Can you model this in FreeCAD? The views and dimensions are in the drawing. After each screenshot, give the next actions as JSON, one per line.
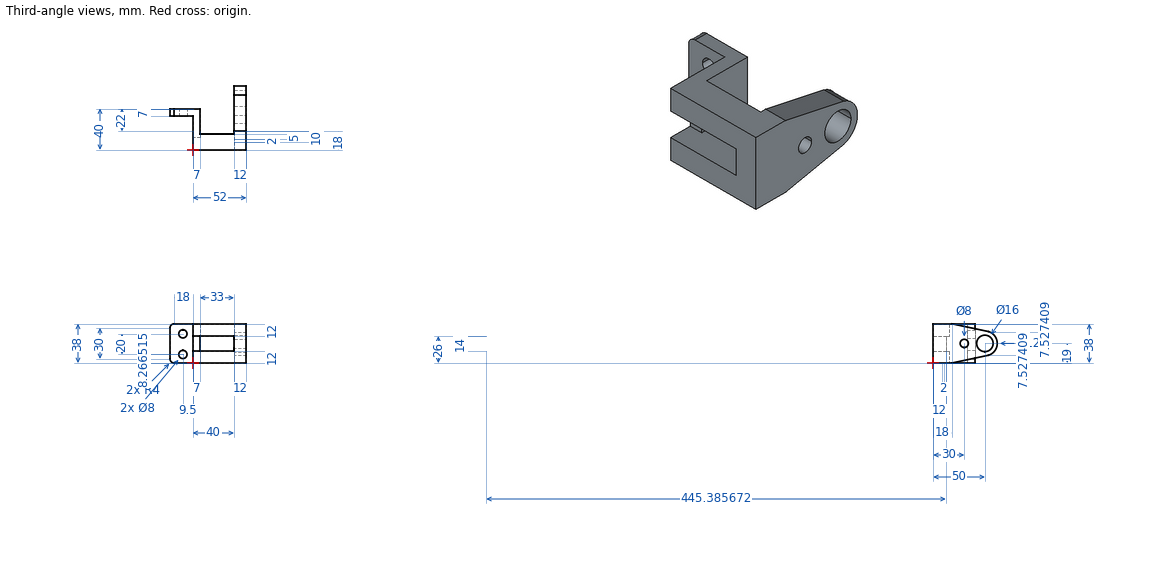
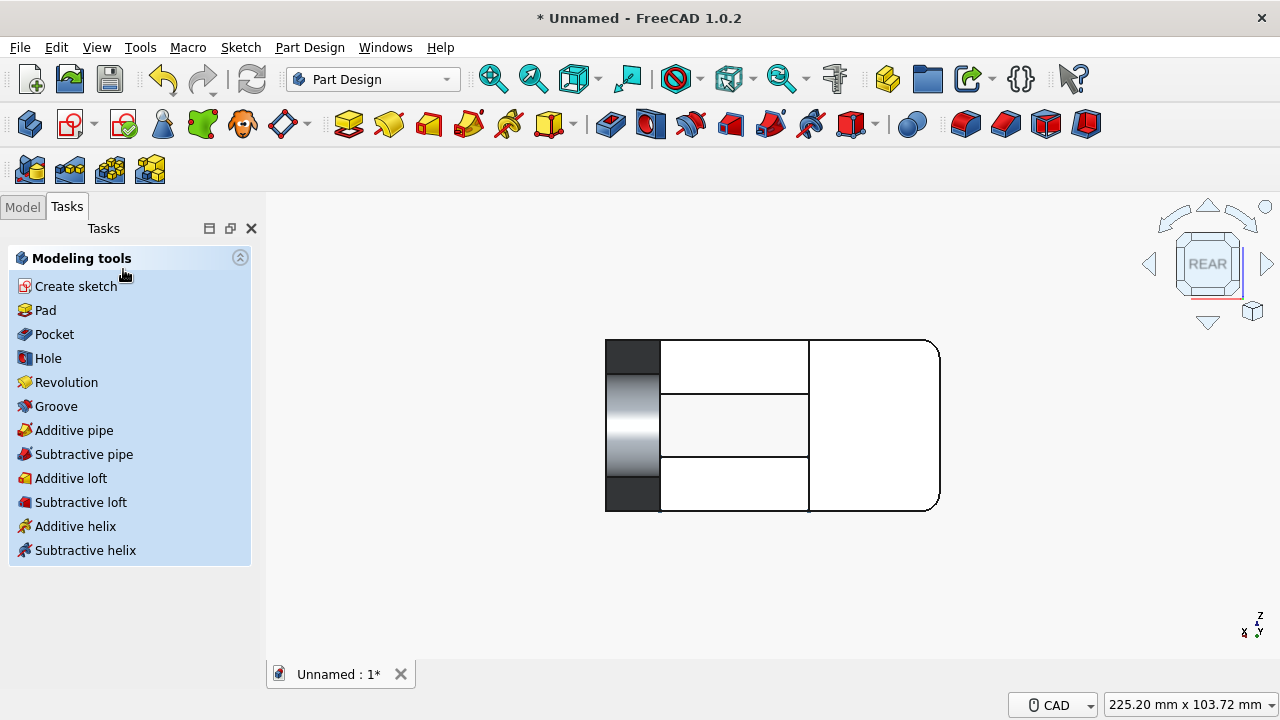
{"action": "left_click", "coordinate": [350, 124]}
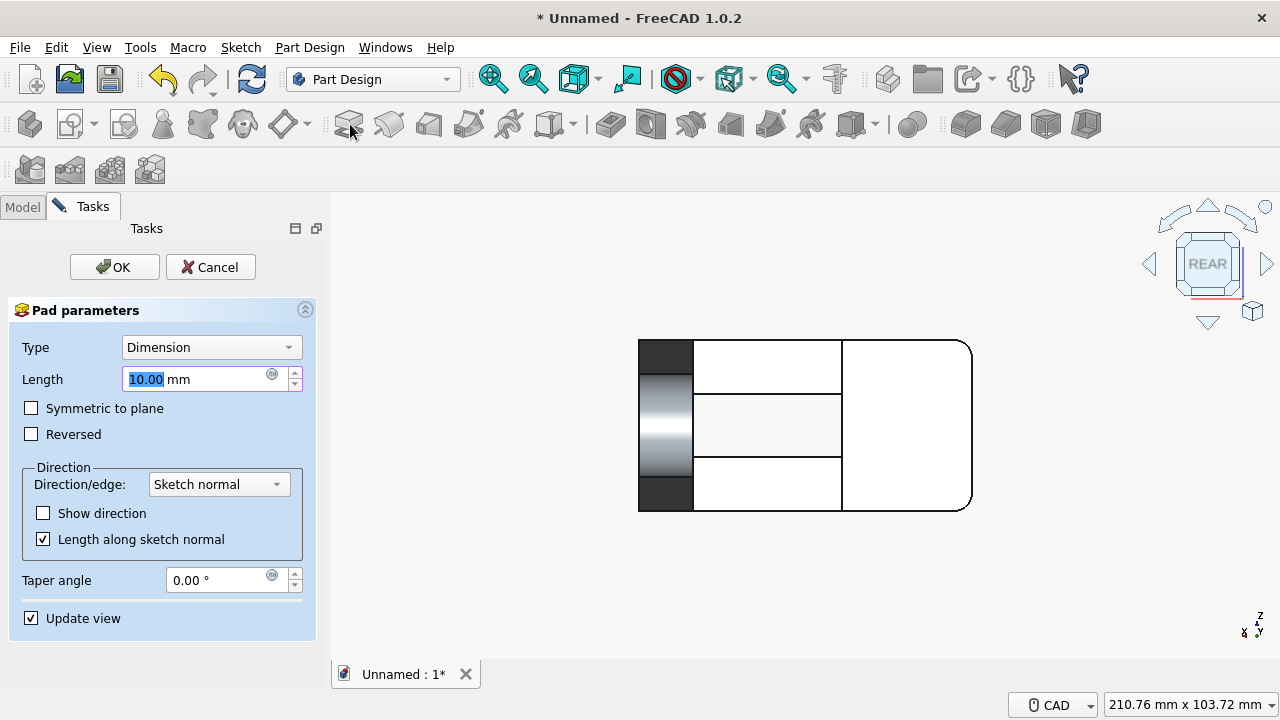
{"action": "type", "text": "2"}
{"action": "key", "text": "Tab"}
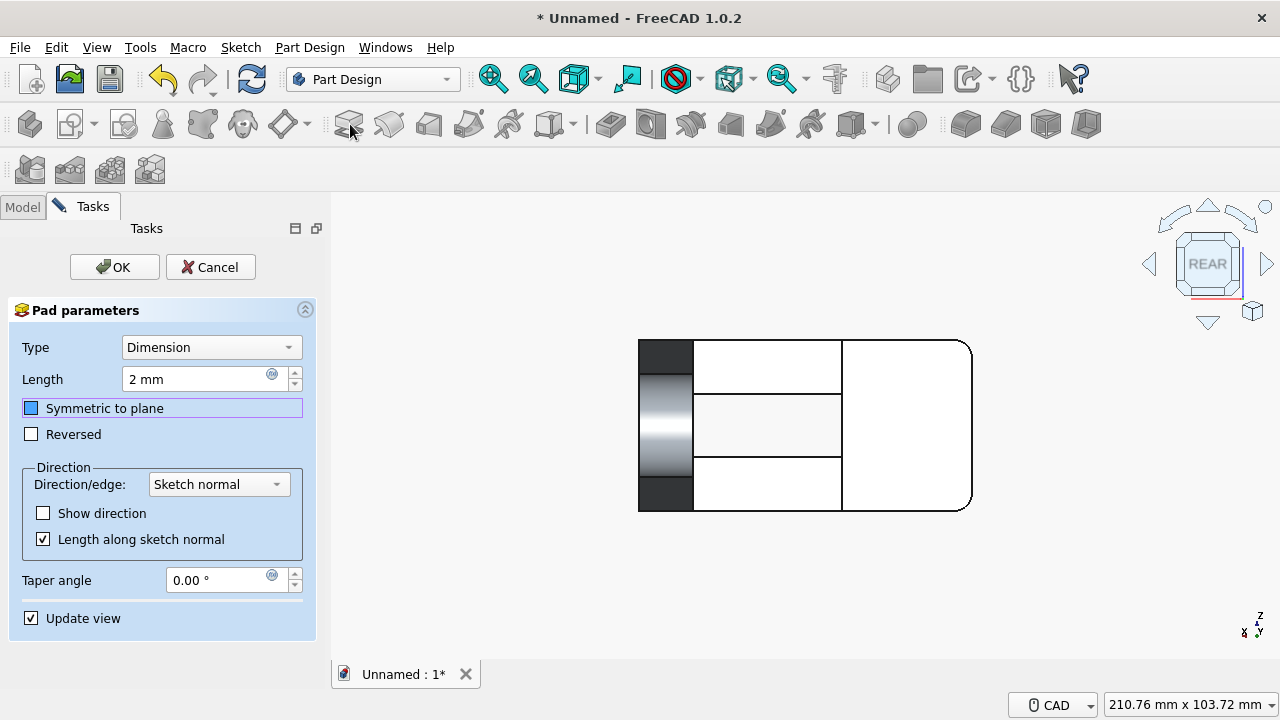
{"action": "left_click", "coordinate": [115, 267]}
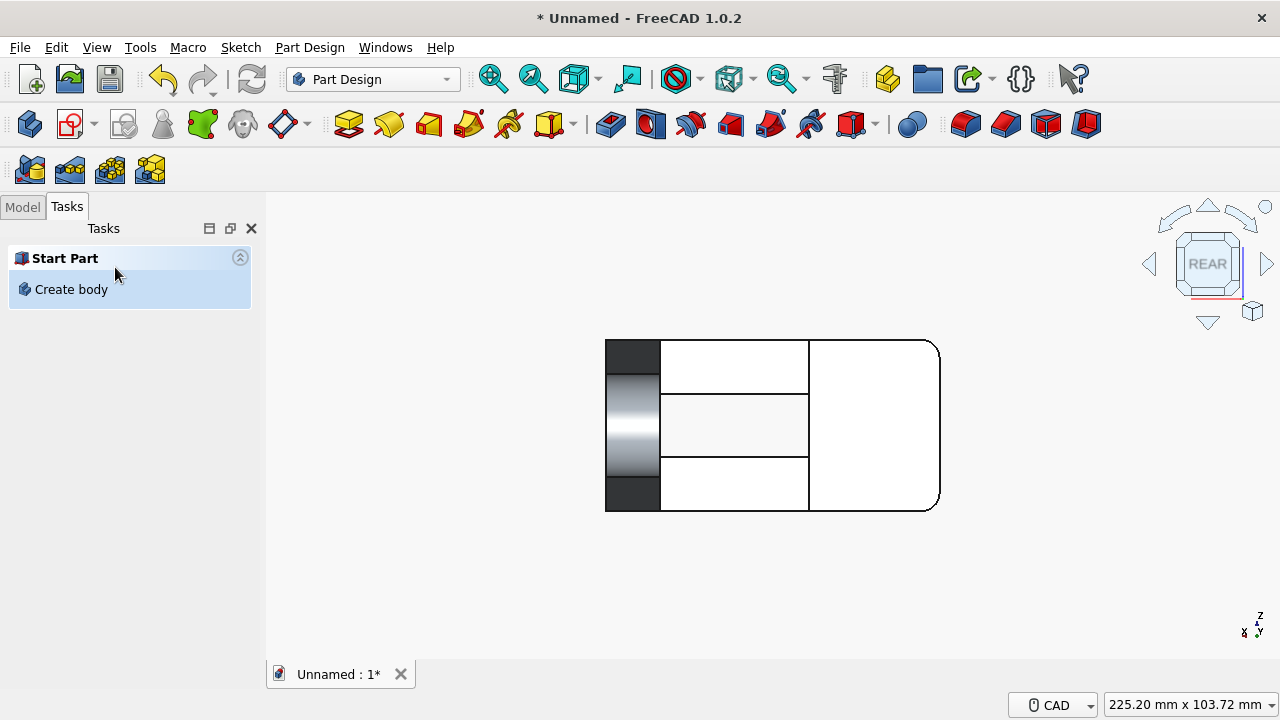
{"action": "left_click", "coordinate": [494, 80]}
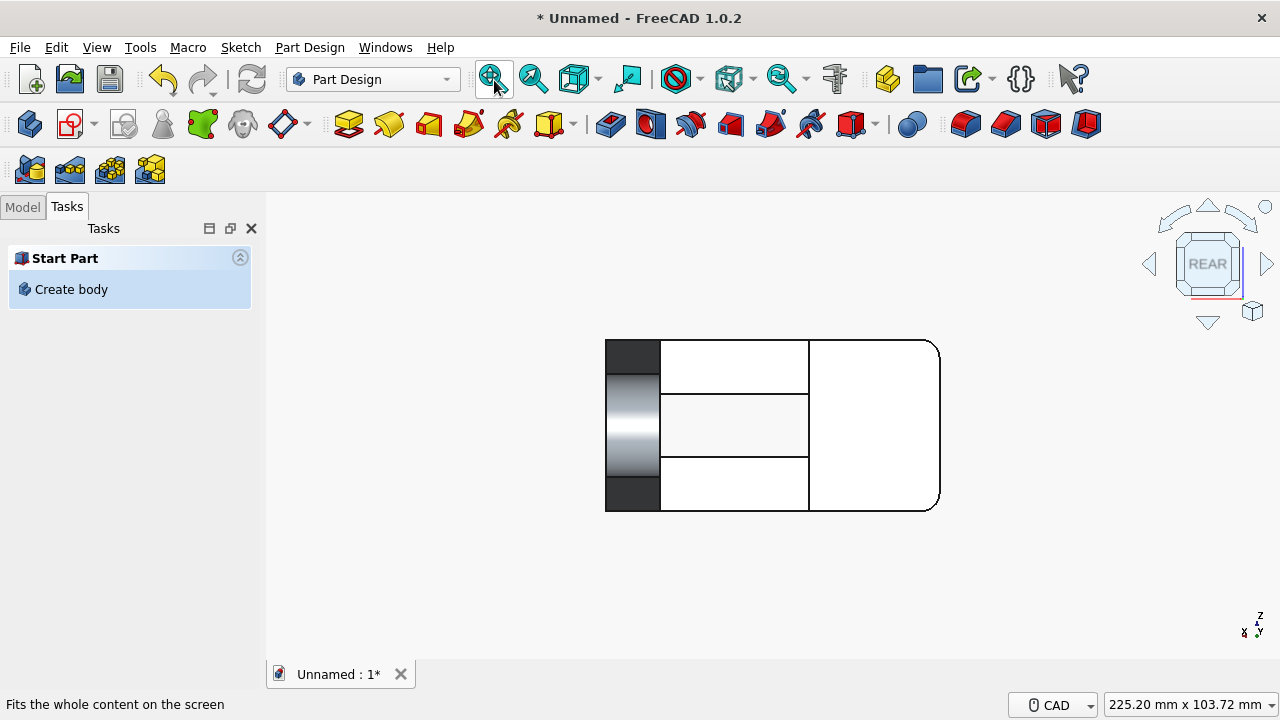
{"action": "left_click", "coordinate": [874, 424]}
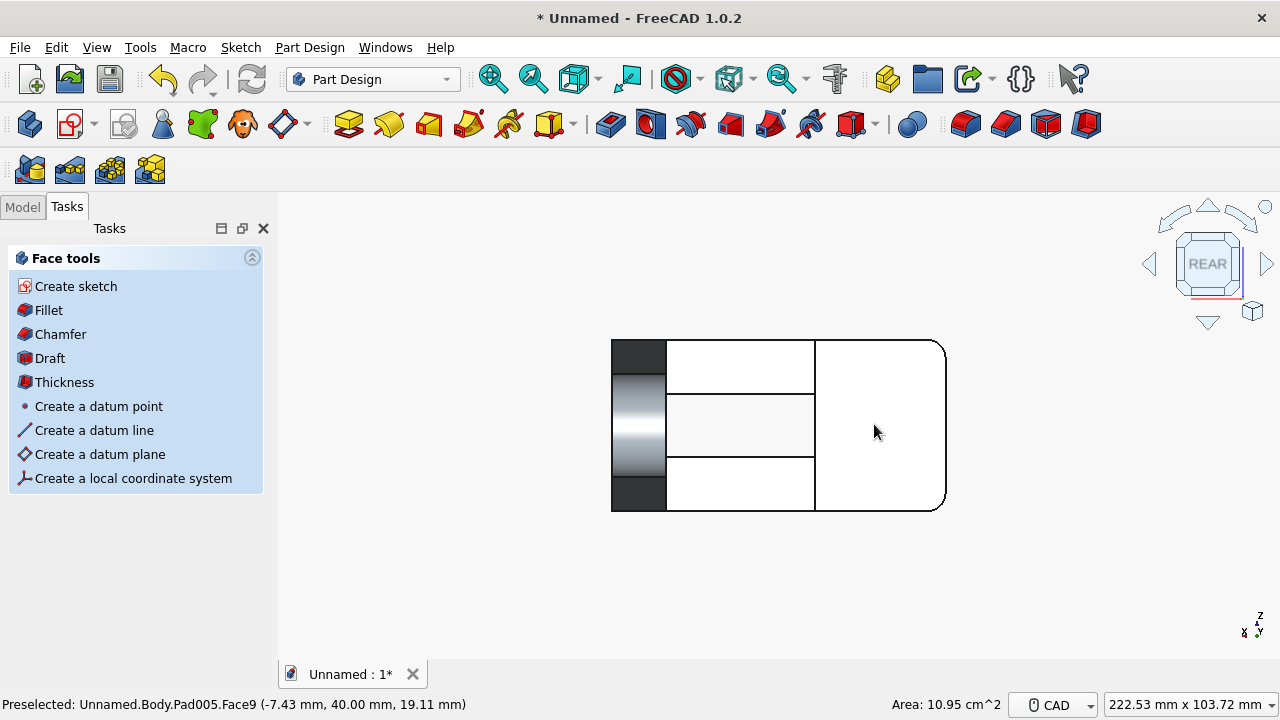
{"action": "left_click", "coordinate": [70, 124]}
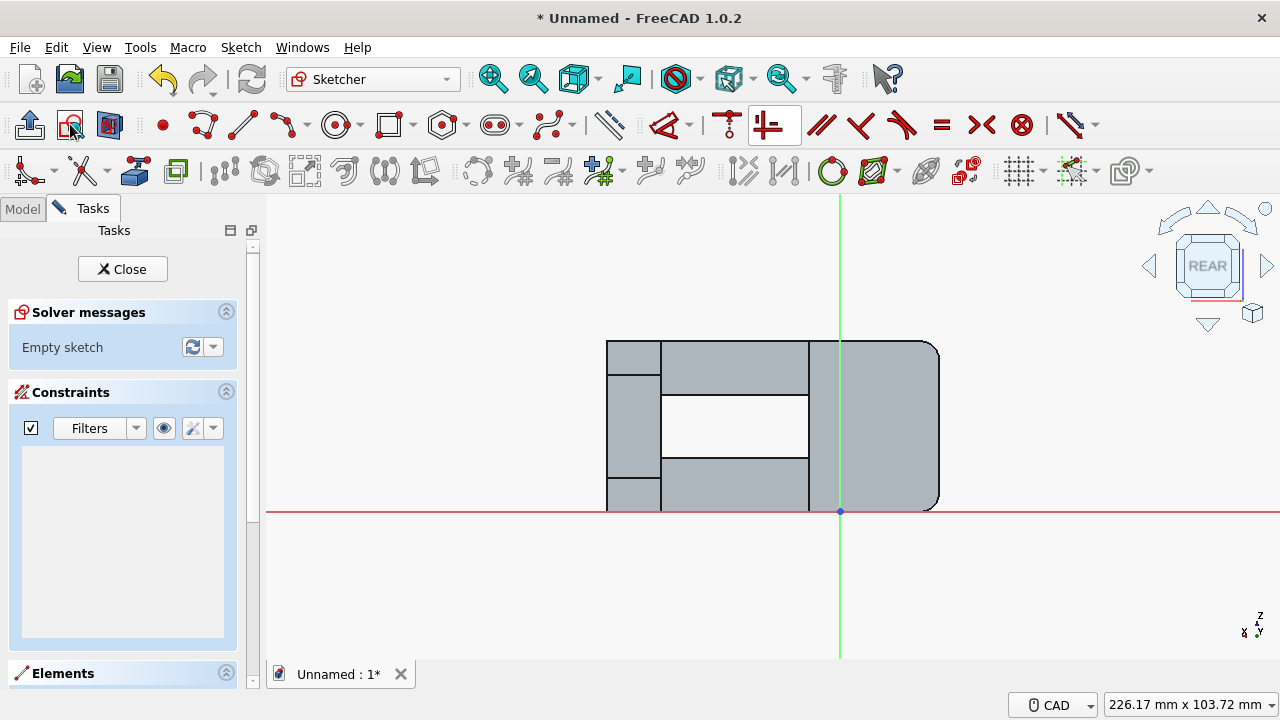
{"action": "left_click", "coordinate": [110, 126]}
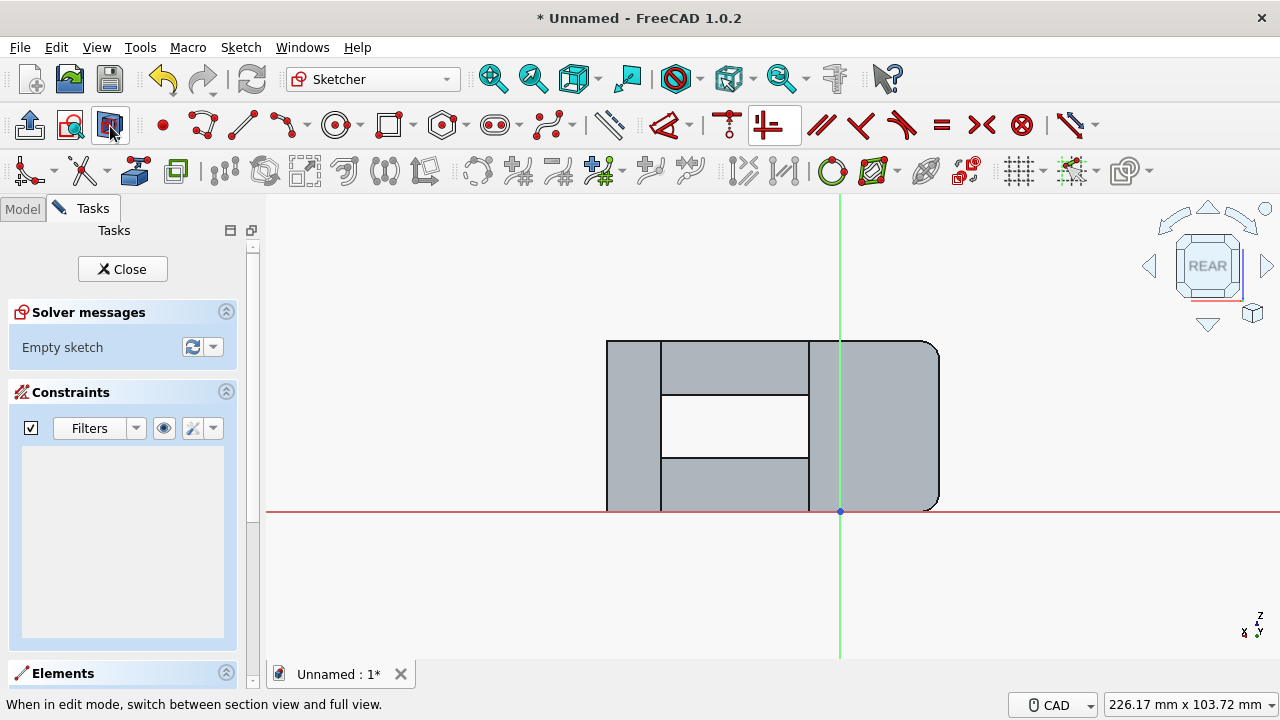
{"action": "scroll", "coordinate": [1072, 455], "scroll_direction": "up", "scroll_amount": 3}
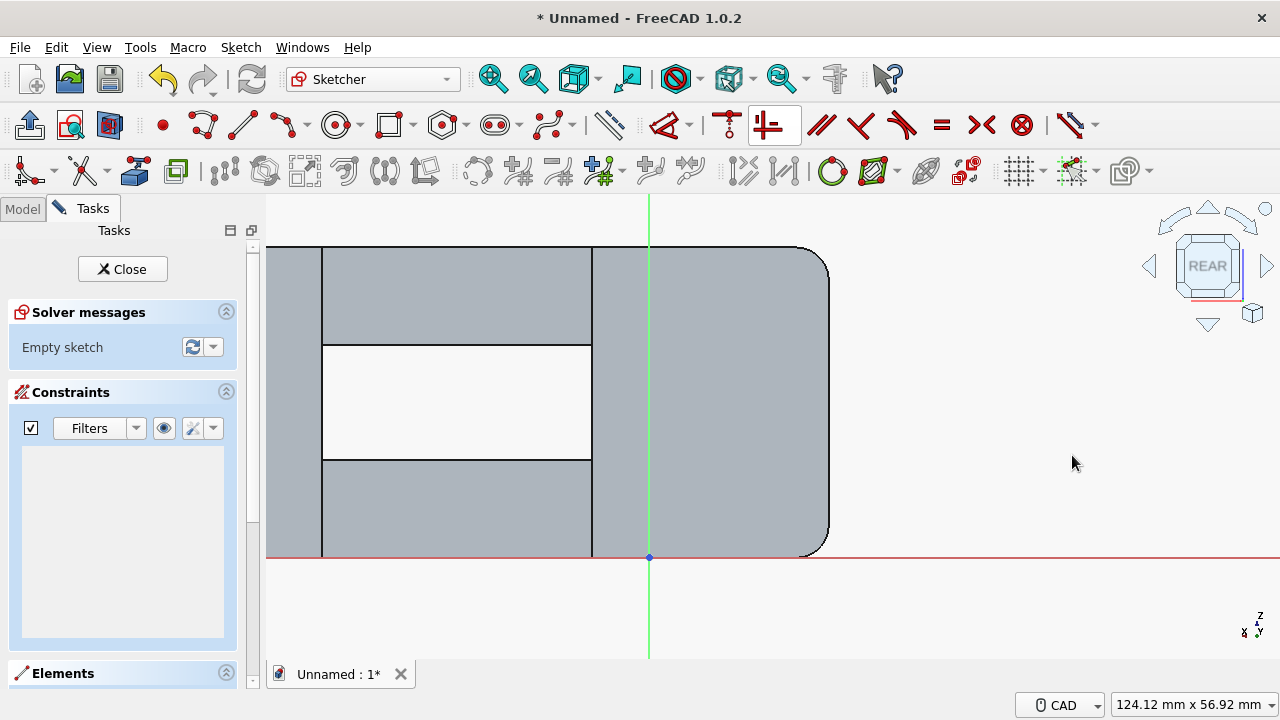
{"action": "left_click", "coordinate": [336, 126]}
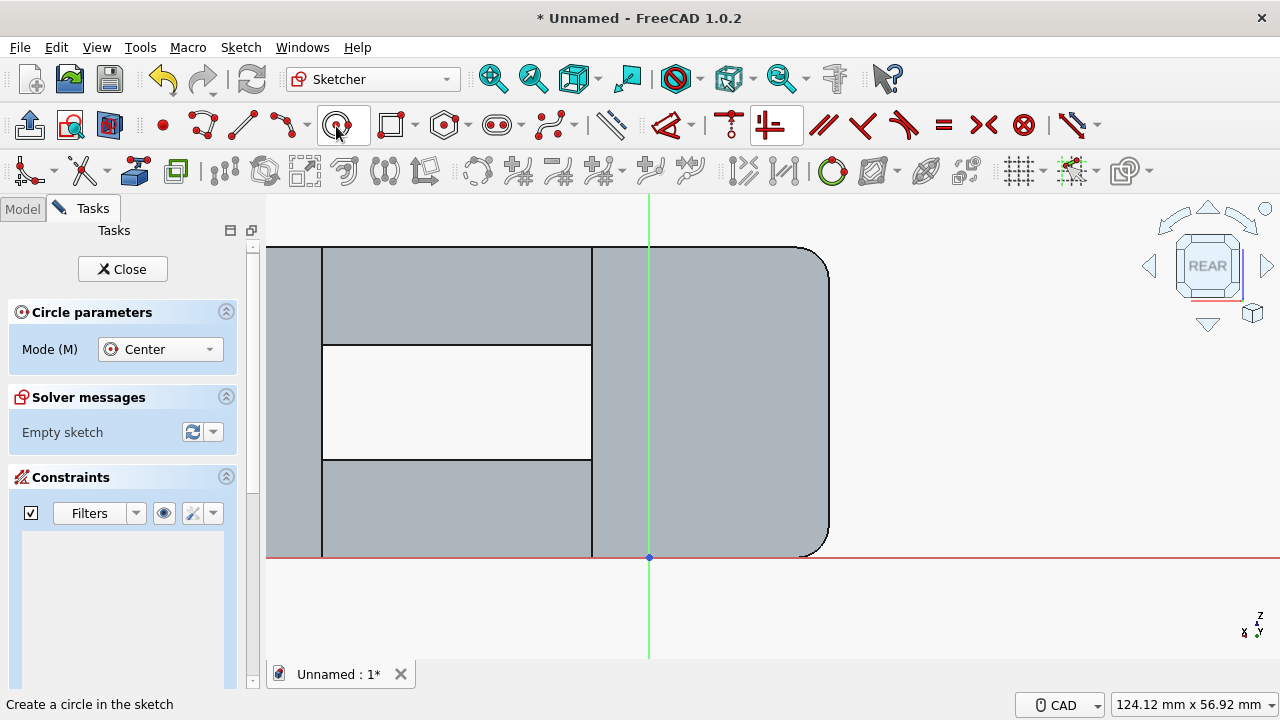
{"action": "left_click", "coordinate": [727, 490]}
{"action": "left_click", "coordinate": [750, 467]}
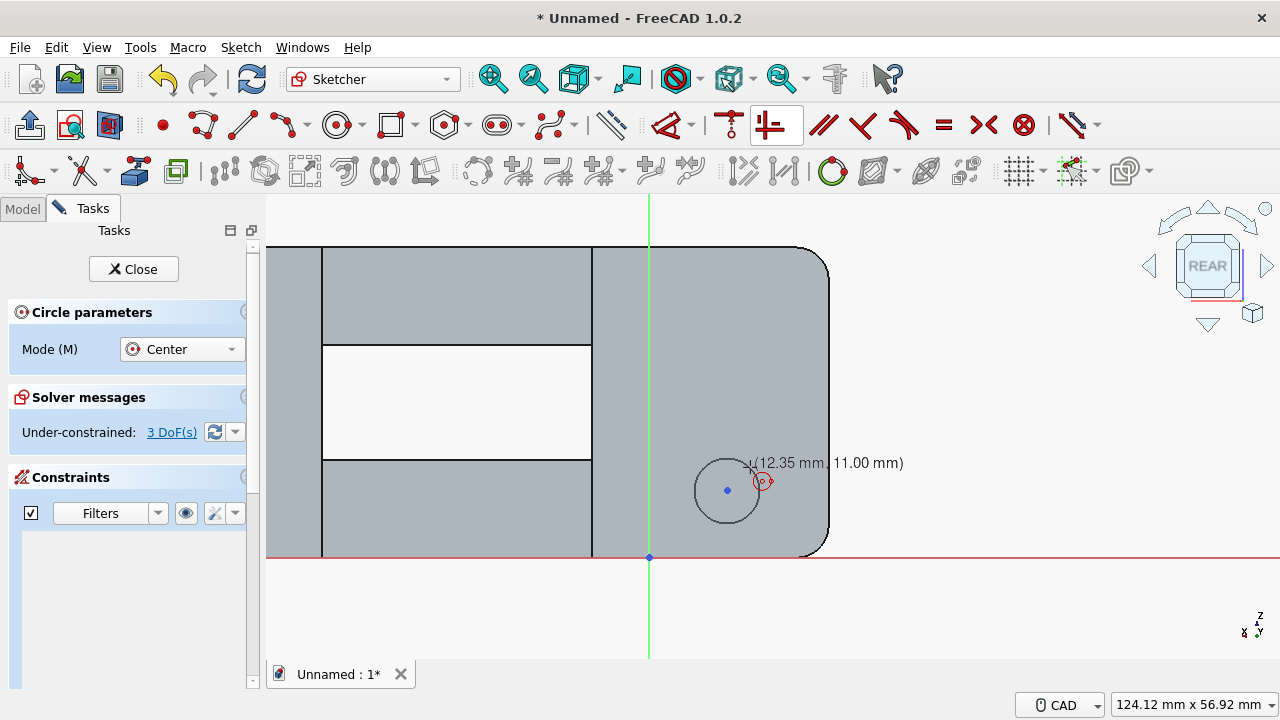
{"action": "left_click", "coordinate": [727, 327]}
{"action": "left_click", "coordinate": [750, 304]}
{"action": "key", "text": "Escape"}